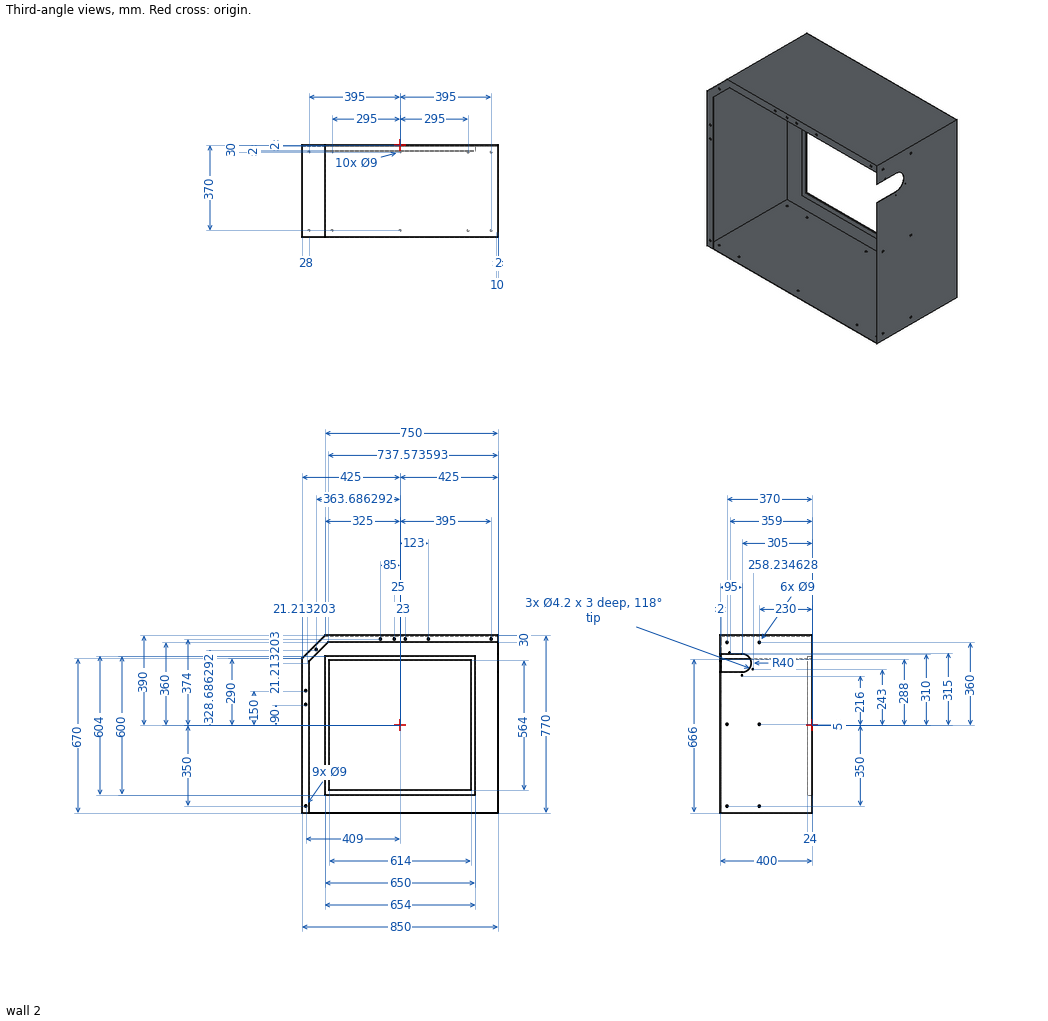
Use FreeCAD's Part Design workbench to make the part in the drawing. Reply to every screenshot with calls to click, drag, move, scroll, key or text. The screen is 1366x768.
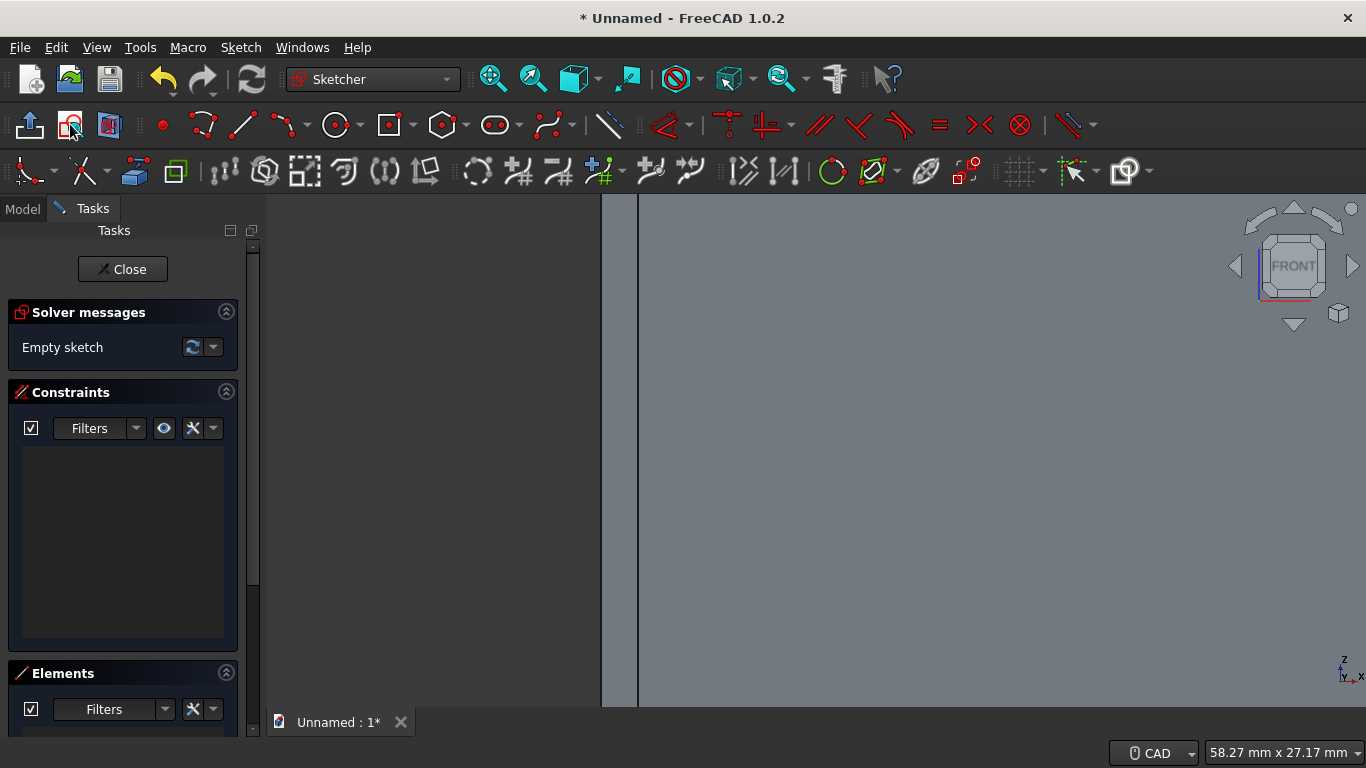
scroll(335, 578, down, 15)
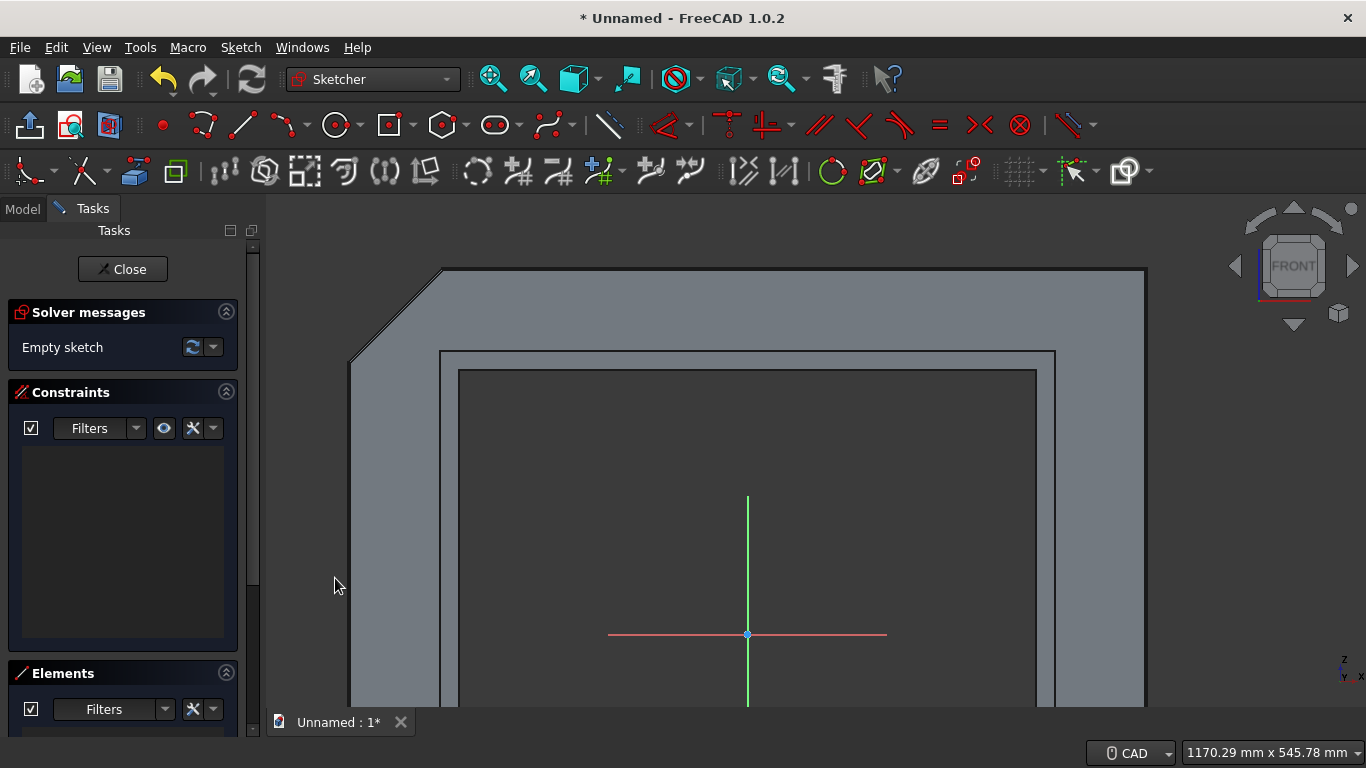
click(204, 126)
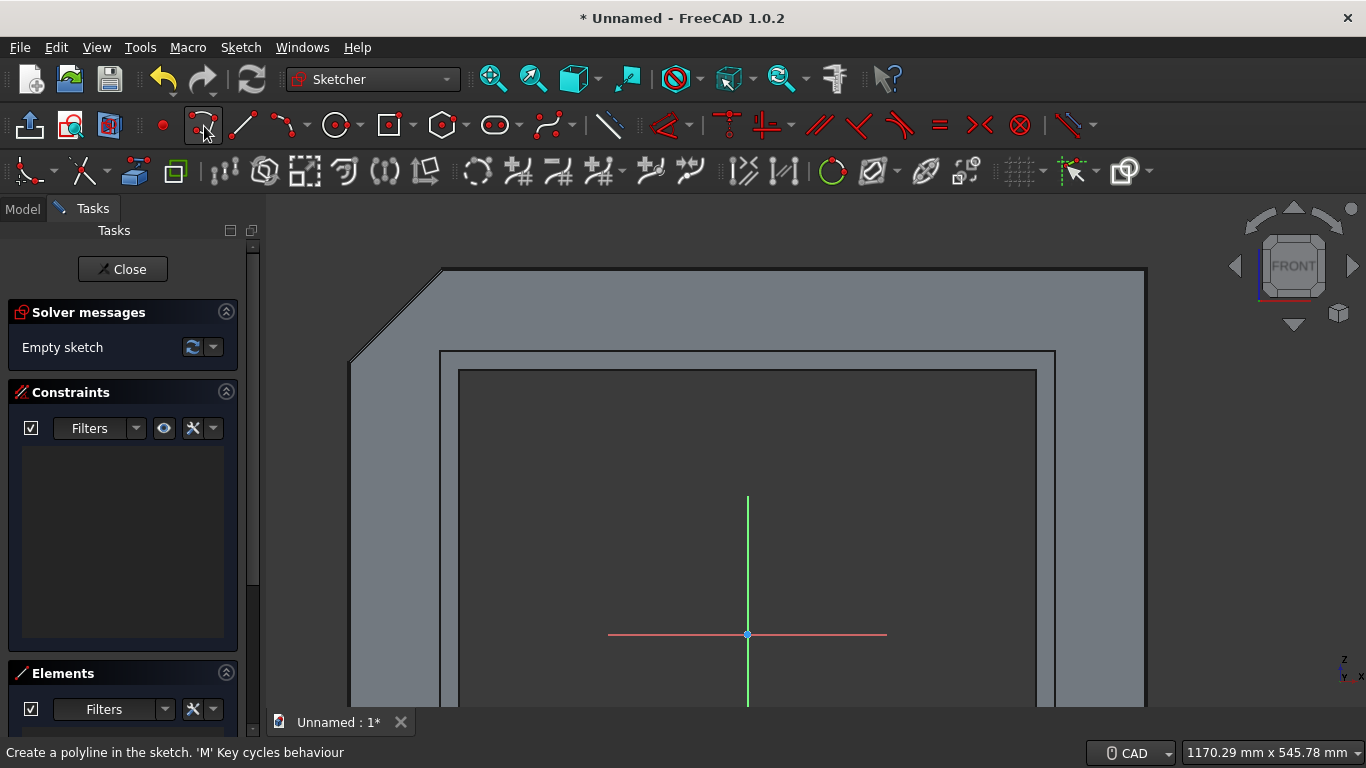
click(454, 297)
click(1147, 297)
click(1147, 268)
click(442, 268)
click(348, 362)
click(368, 382)
click(454, 298)
key(Escape)
key(Escape)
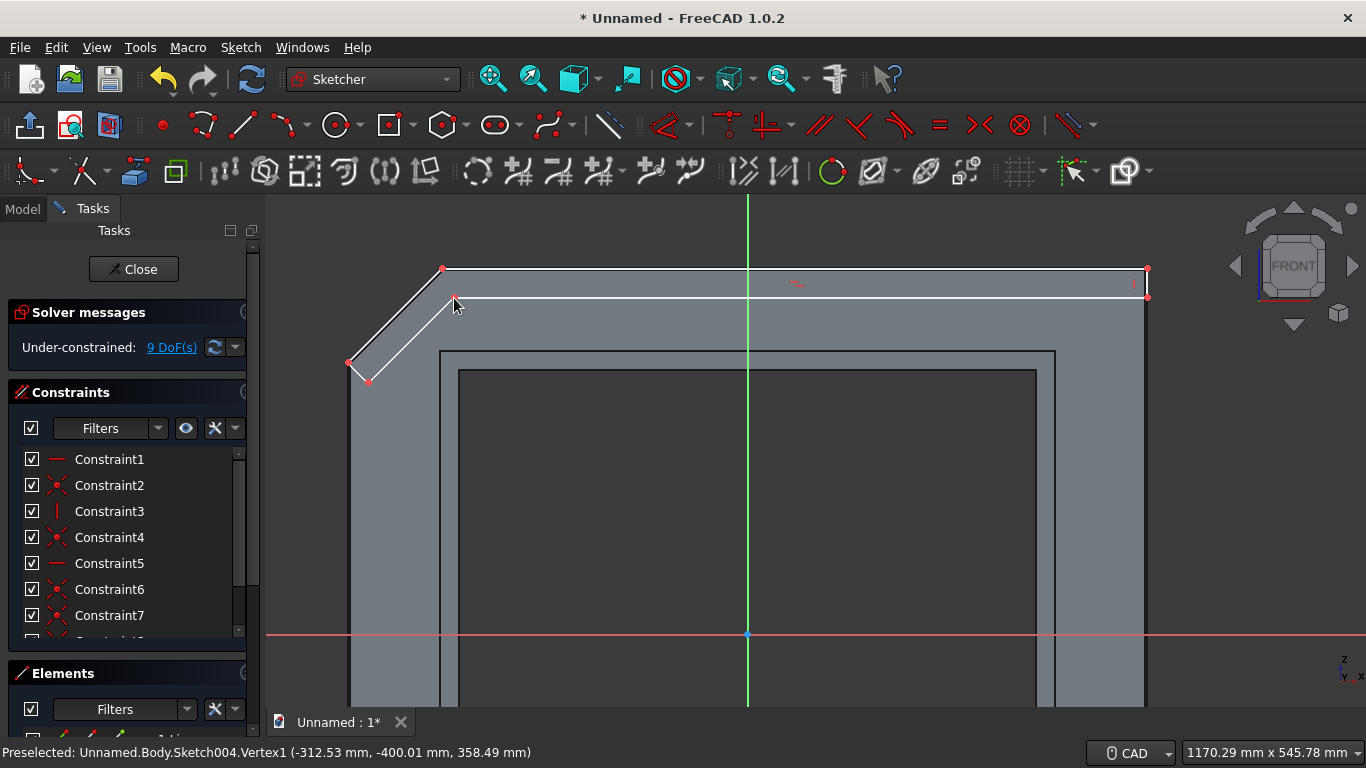
click(664, 126)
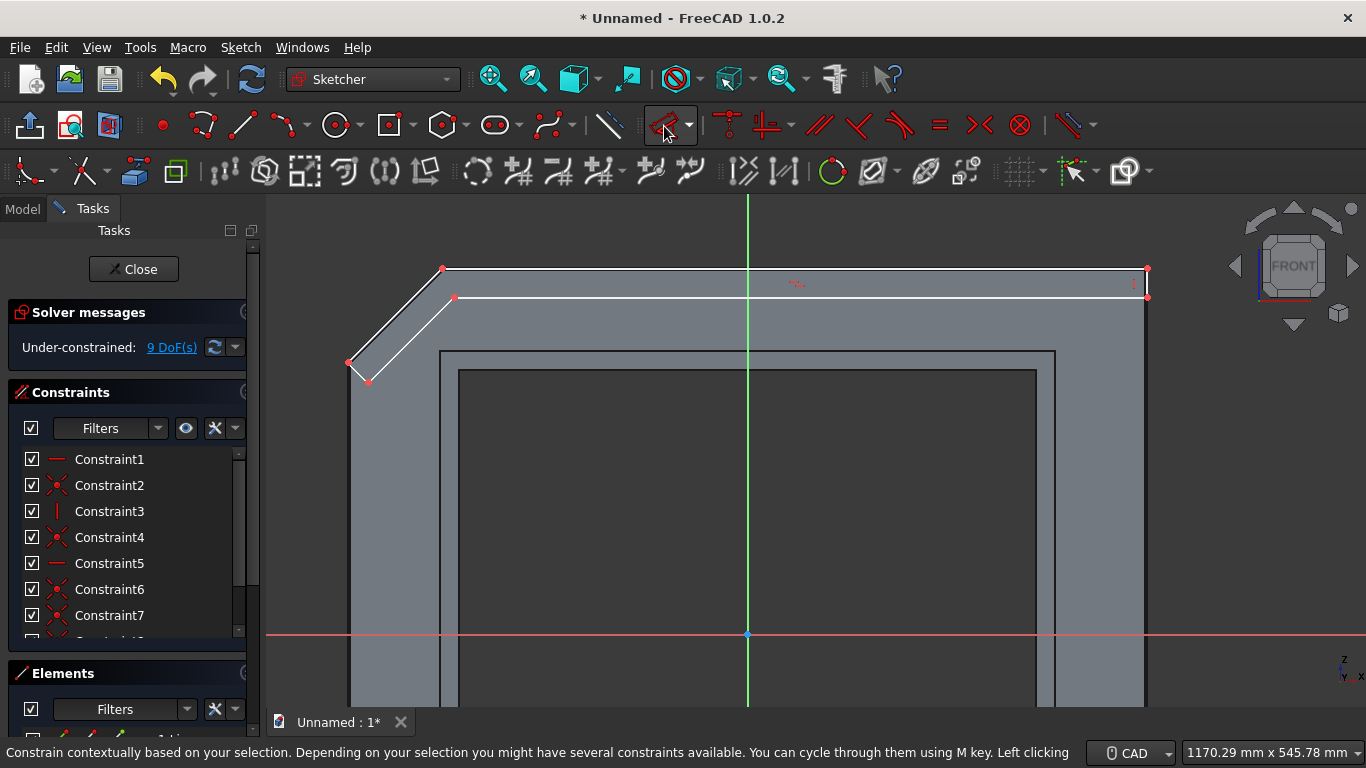
scroll(1147, 286, up, 2)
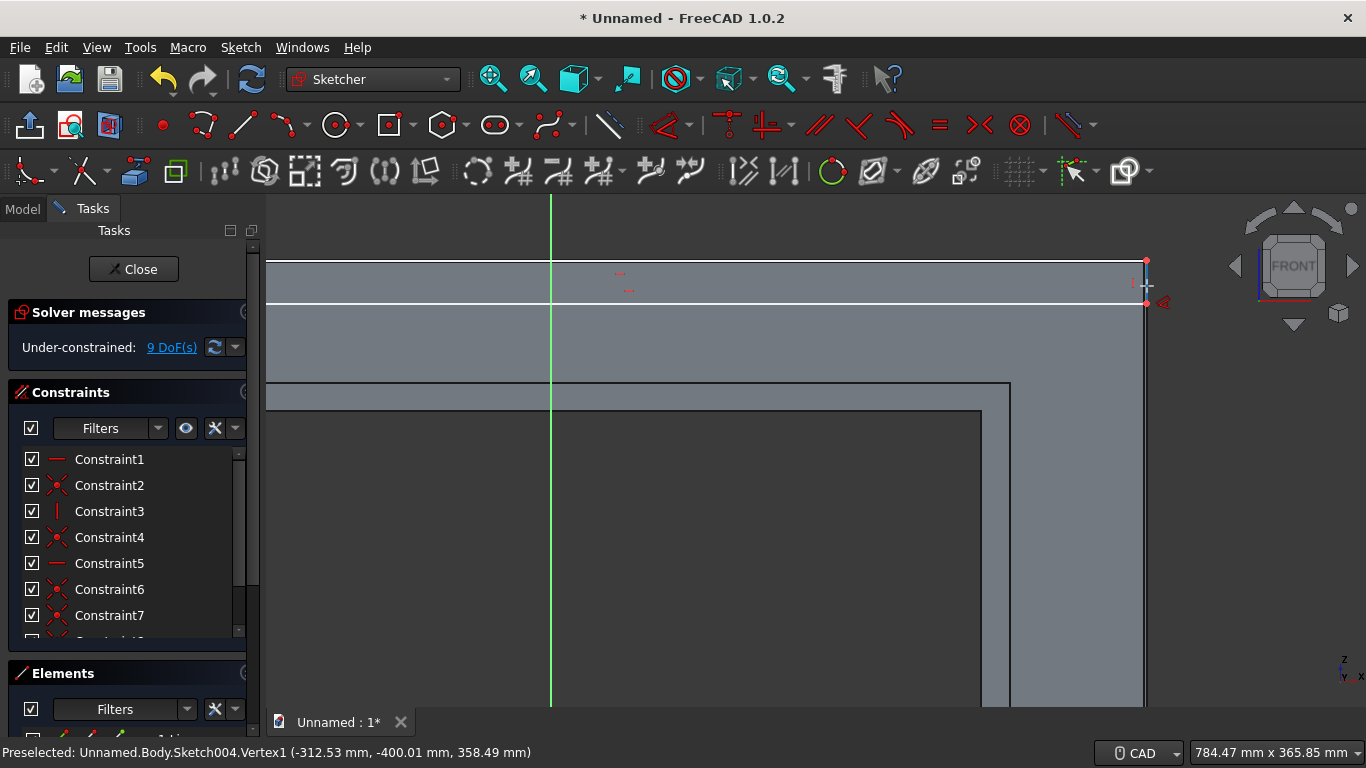
click(1147, 287)
click(1181, 282)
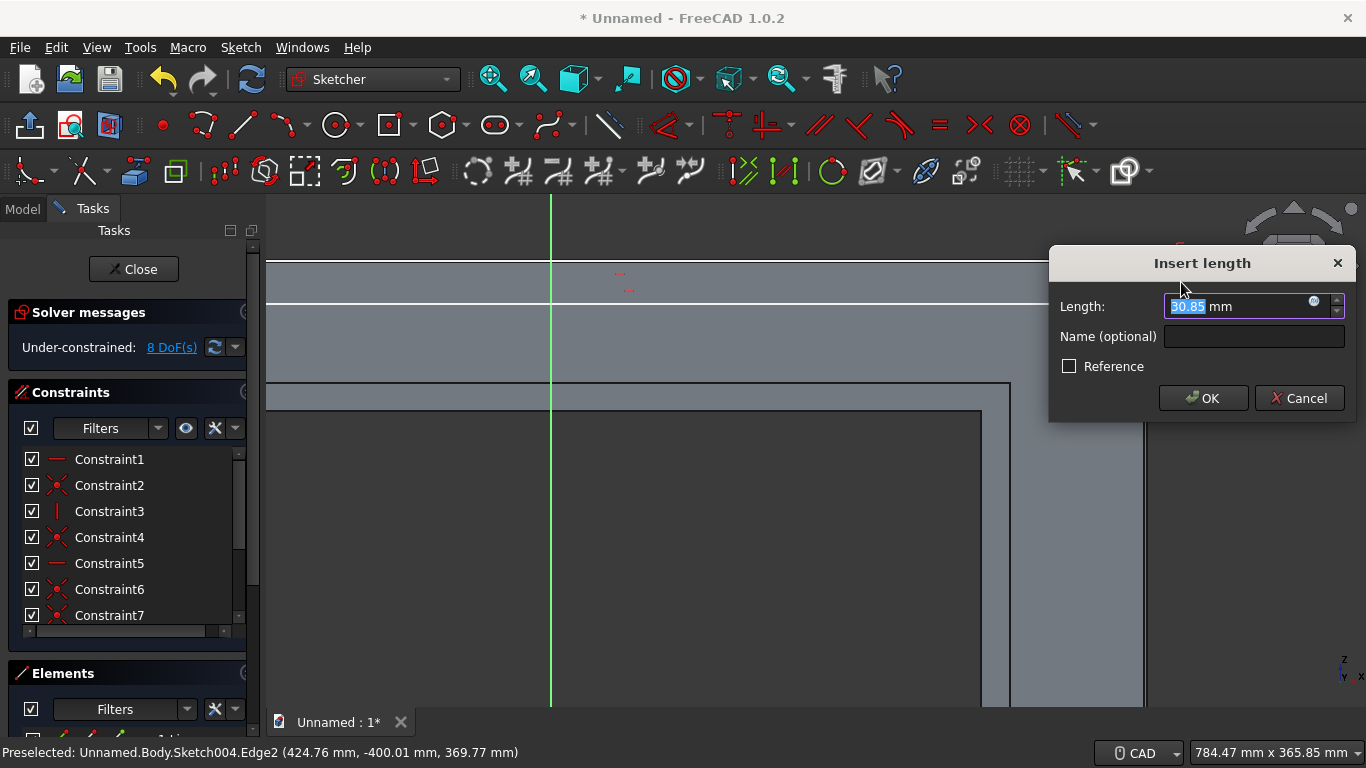
text(30)
key(Return)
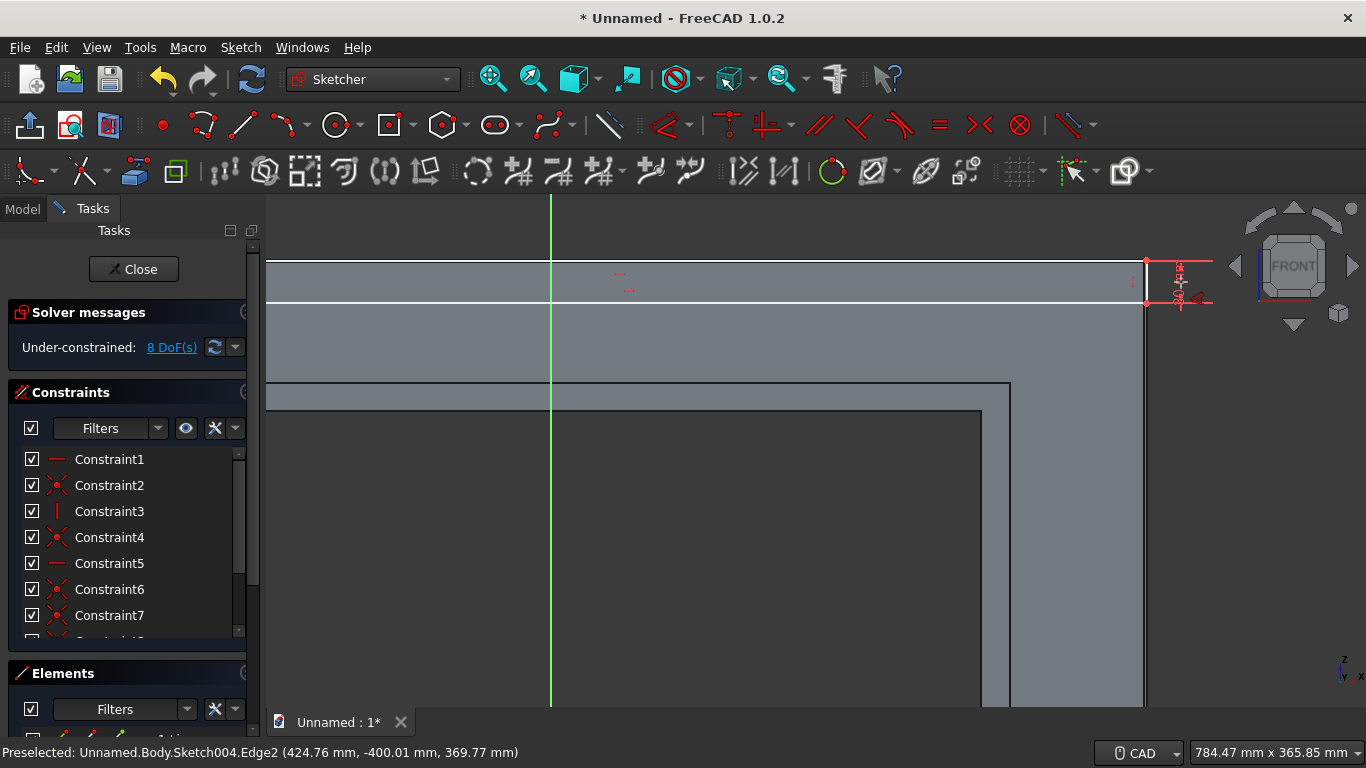
click(831, 261)
click(720, 227)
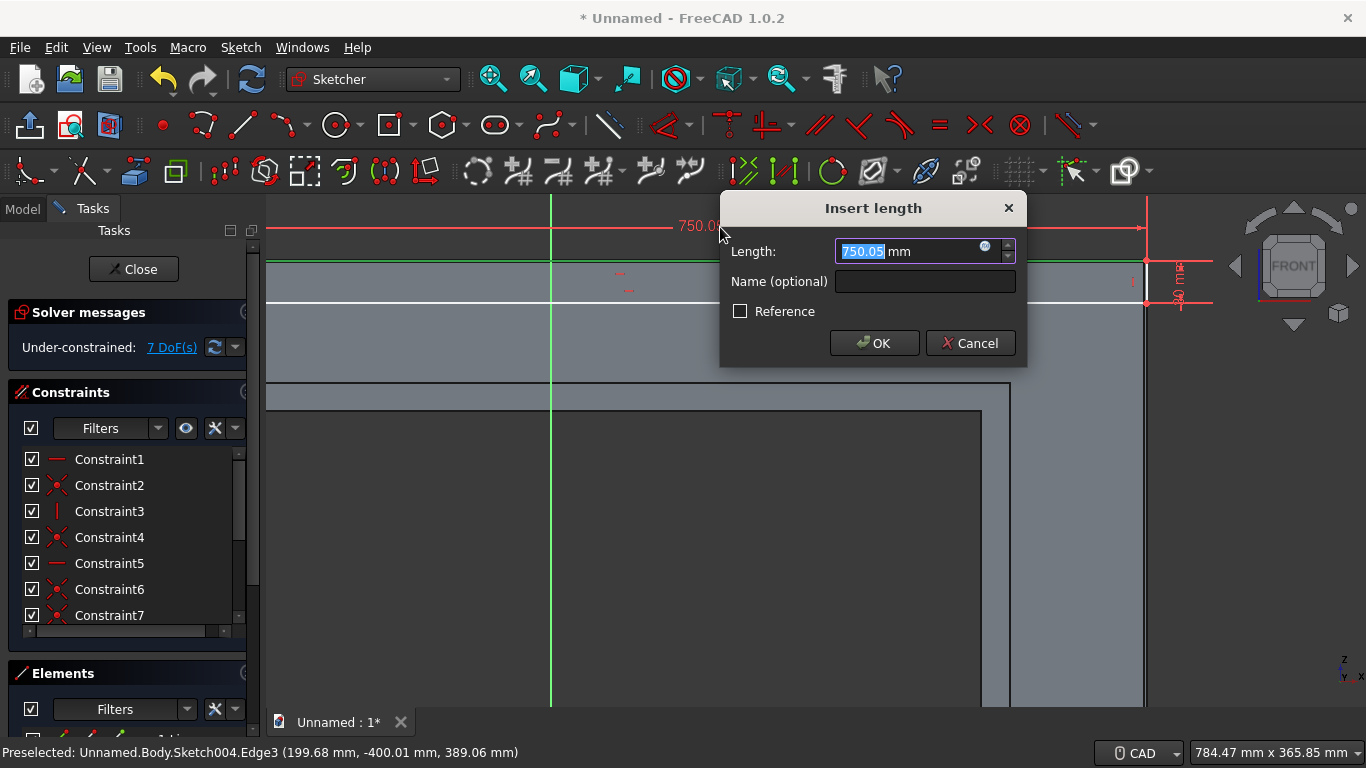
text(750)
key(Return)